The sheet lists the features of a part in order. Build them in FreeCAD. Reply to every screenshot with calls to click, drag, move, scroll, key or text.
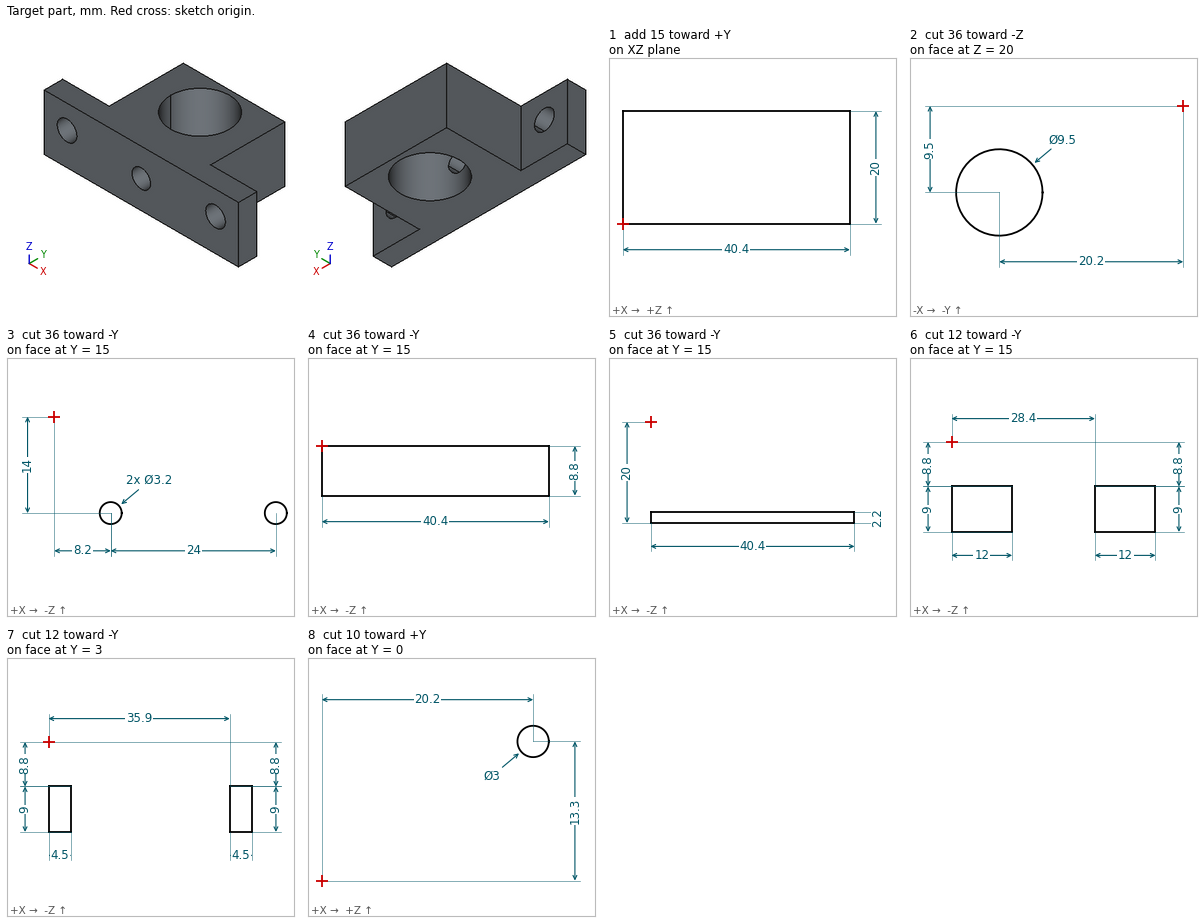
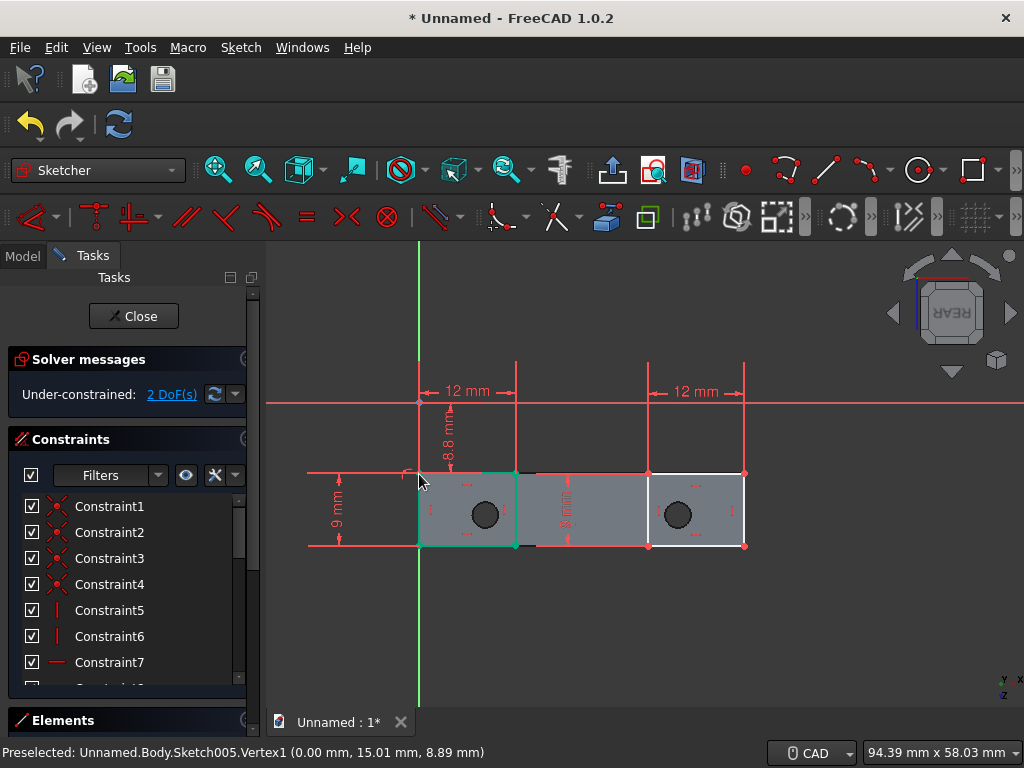
click(648, 474)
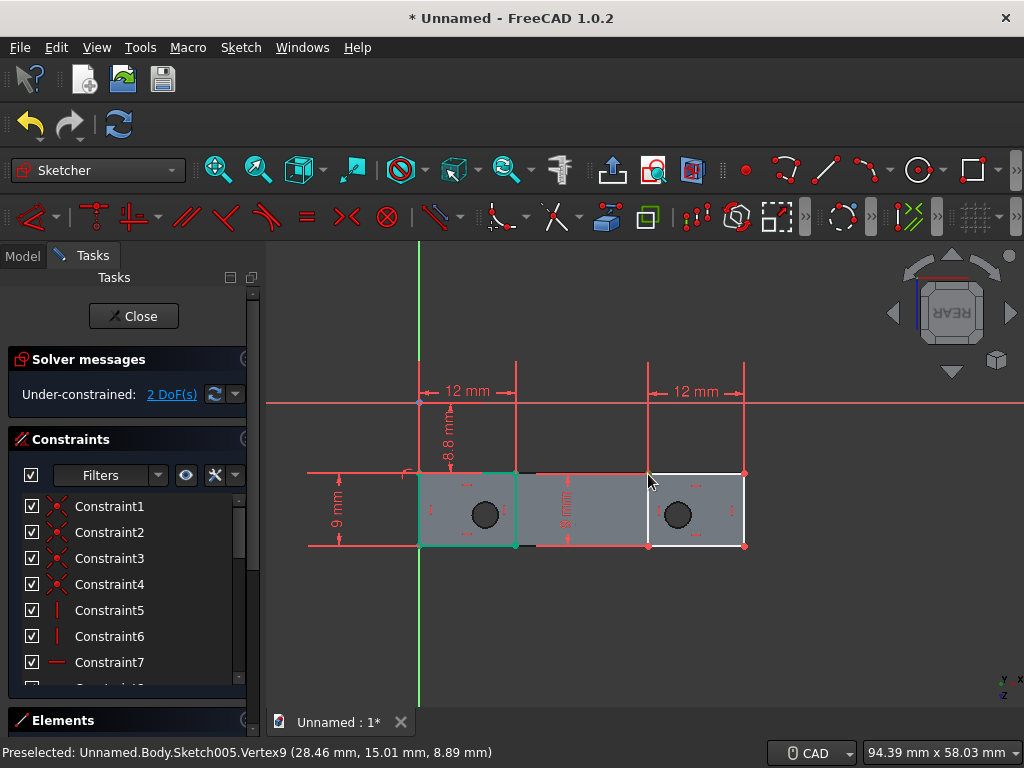
key(i)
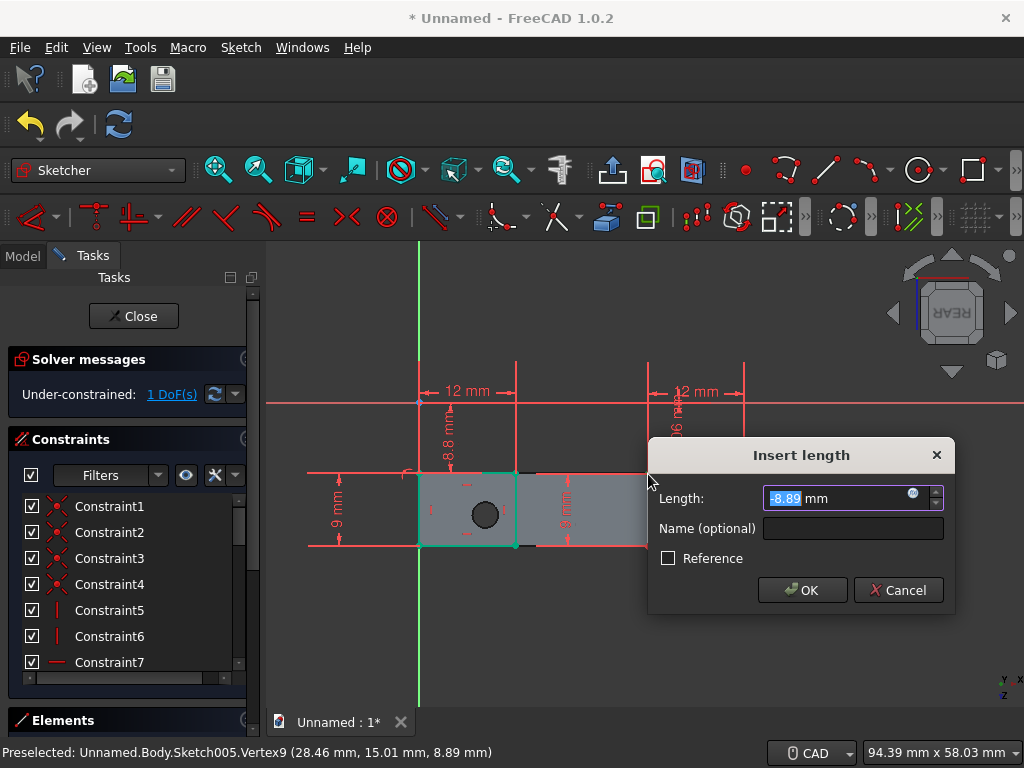
text(-8.8)
key(Return)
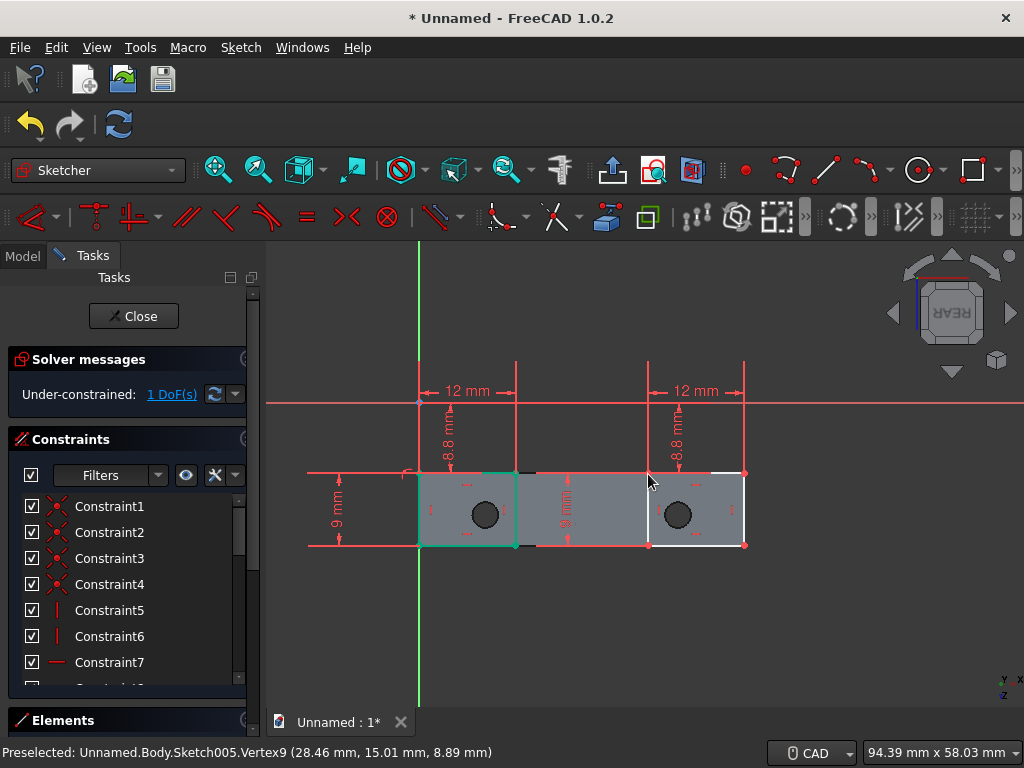
click(648, 473)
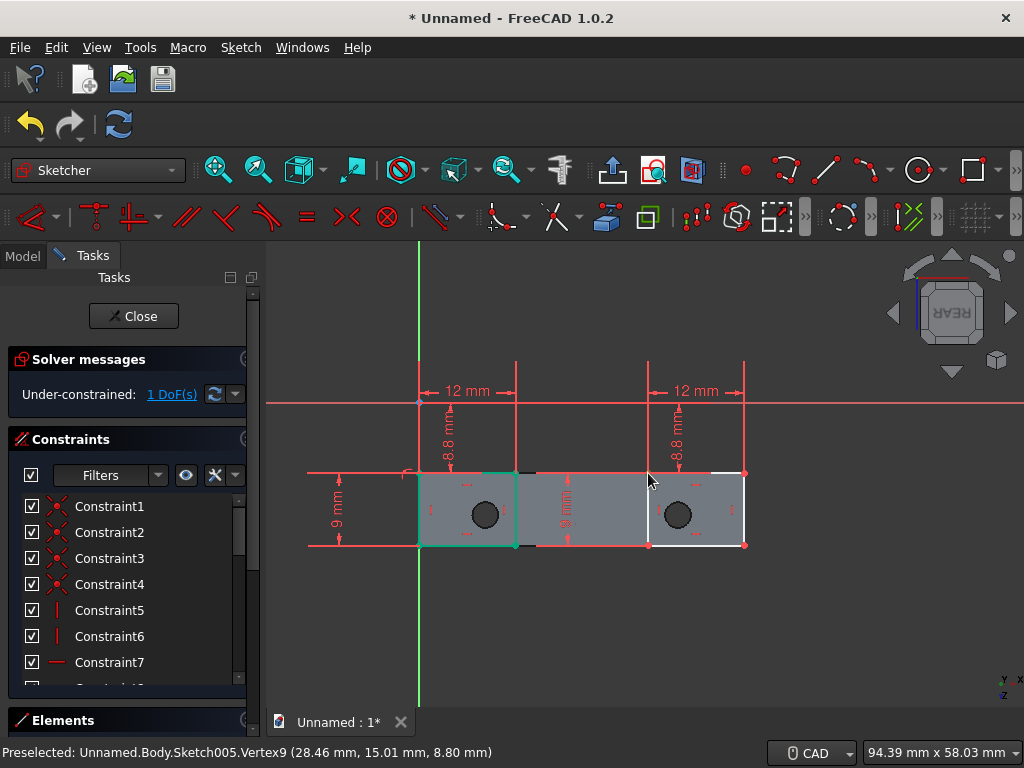
key(l)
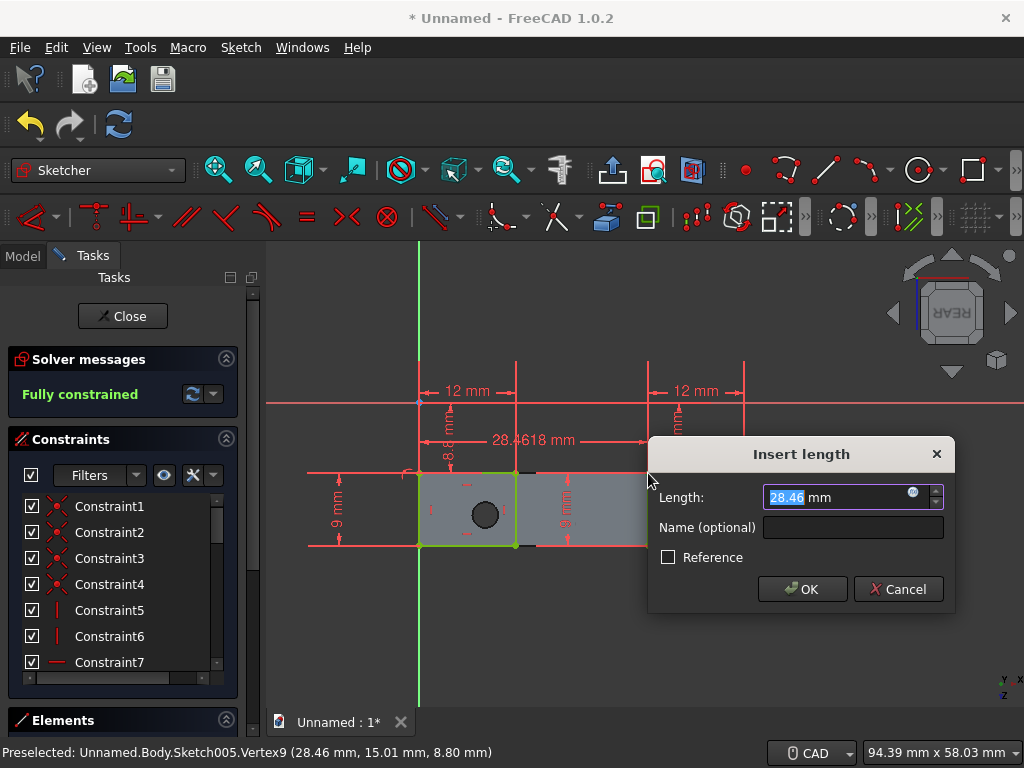
text(28.4)
key(Return)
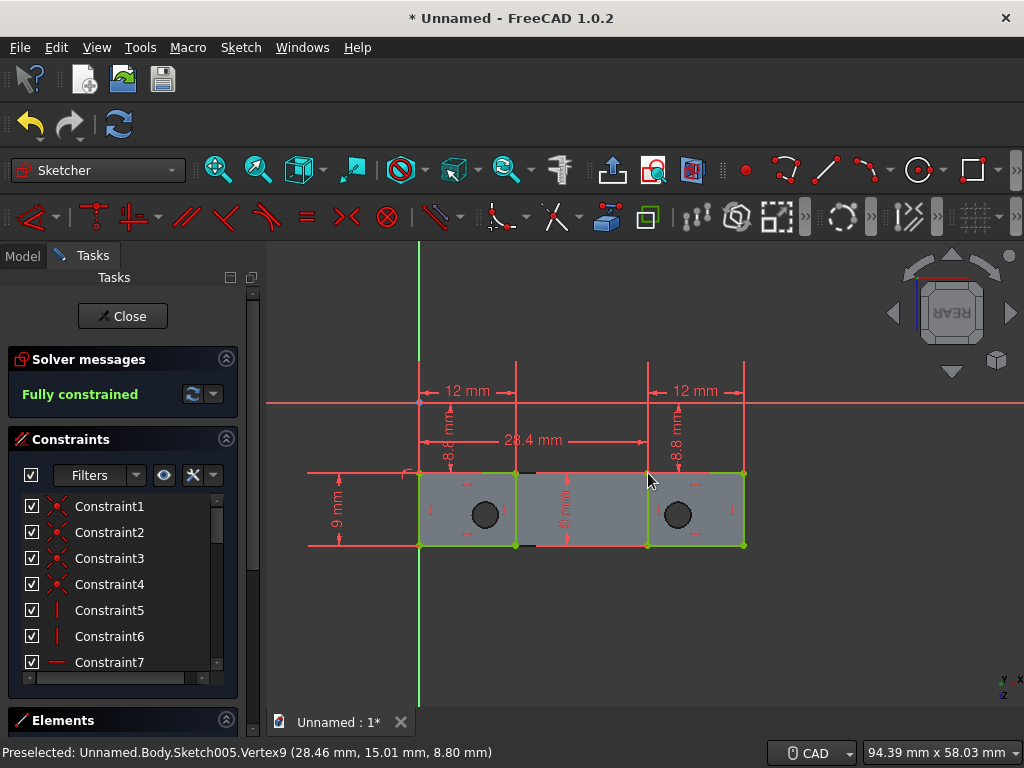
click(123, 316)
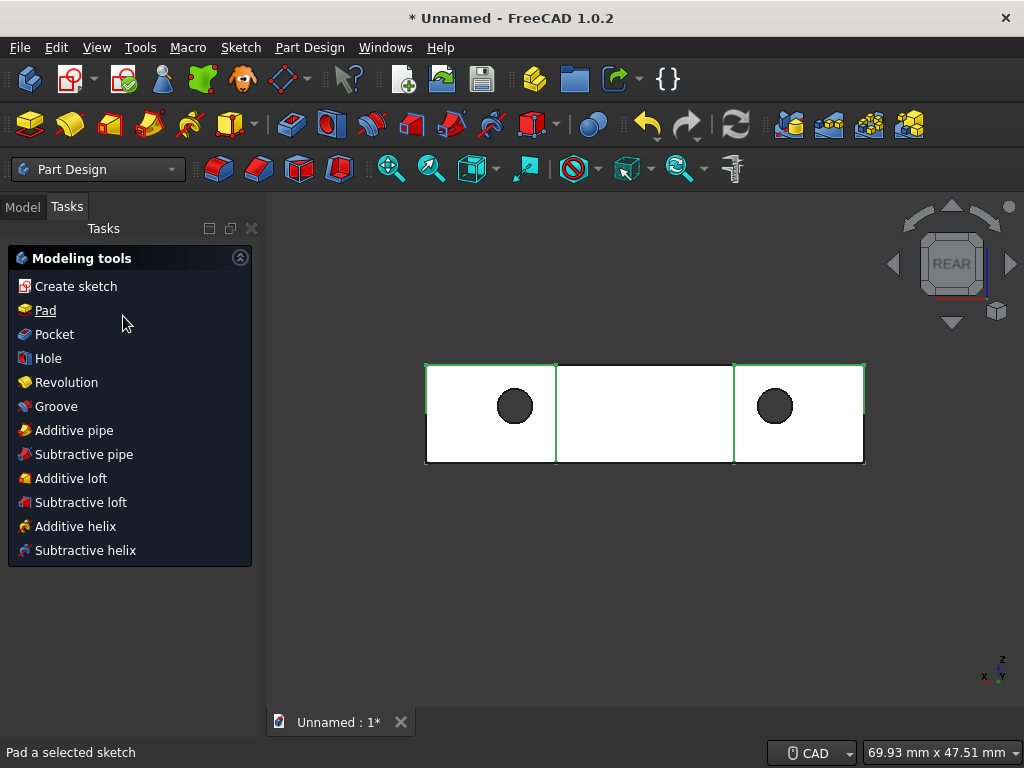
click(292, 124)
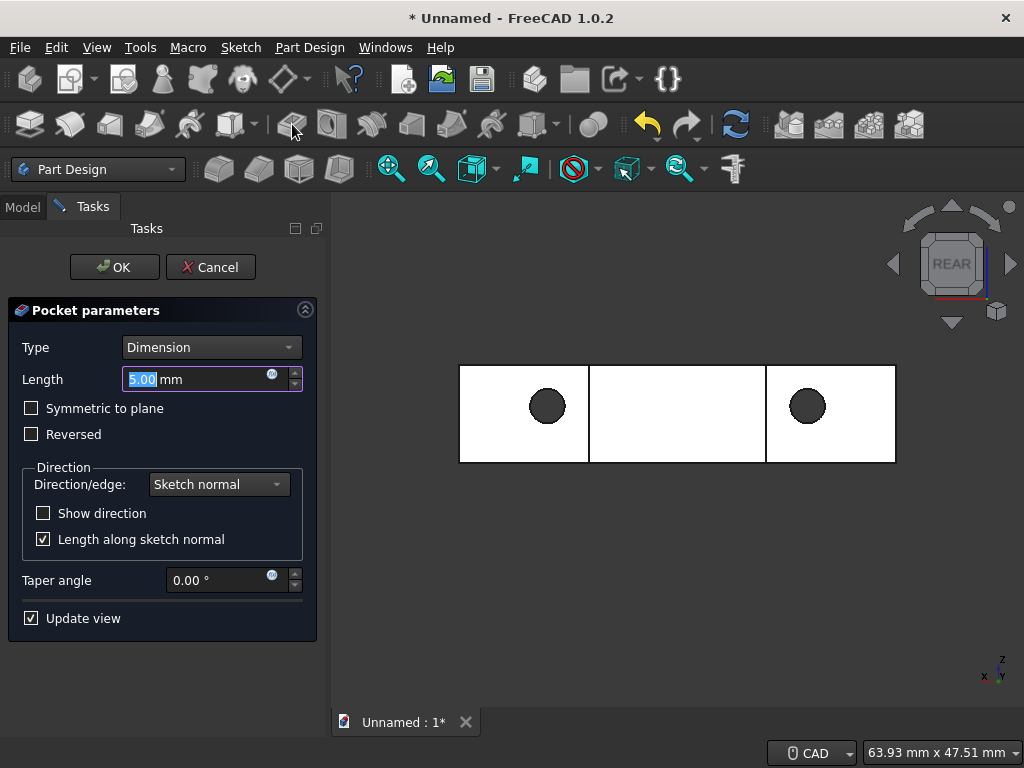
text(12)
key(Tab)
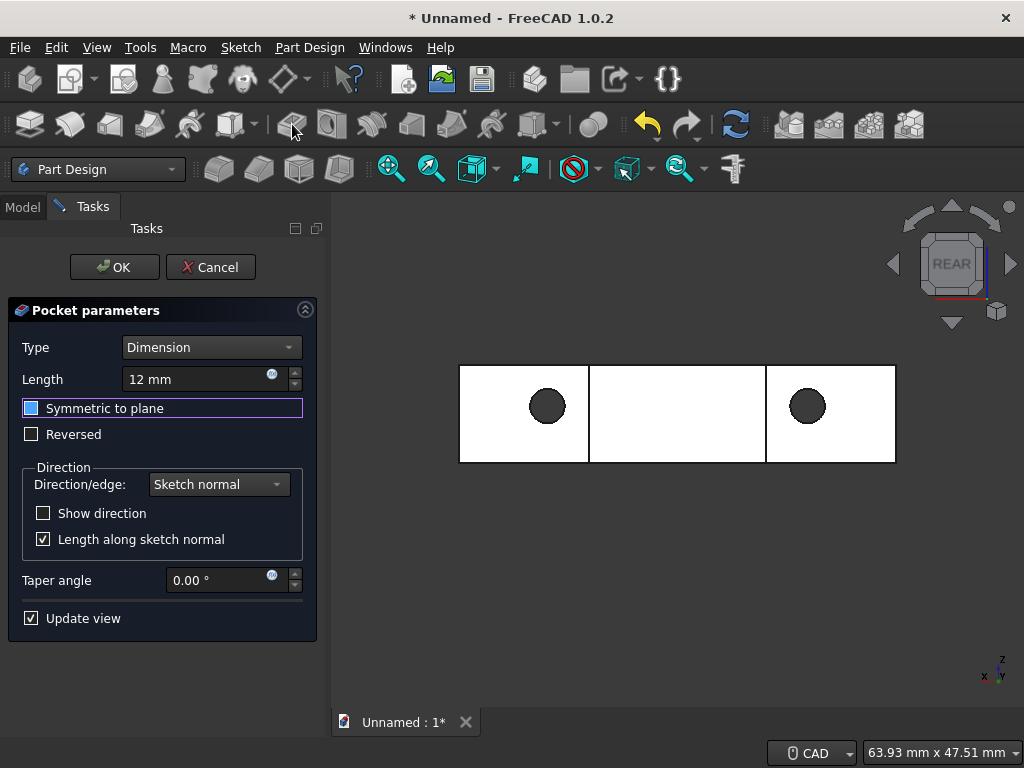
click(115, 267)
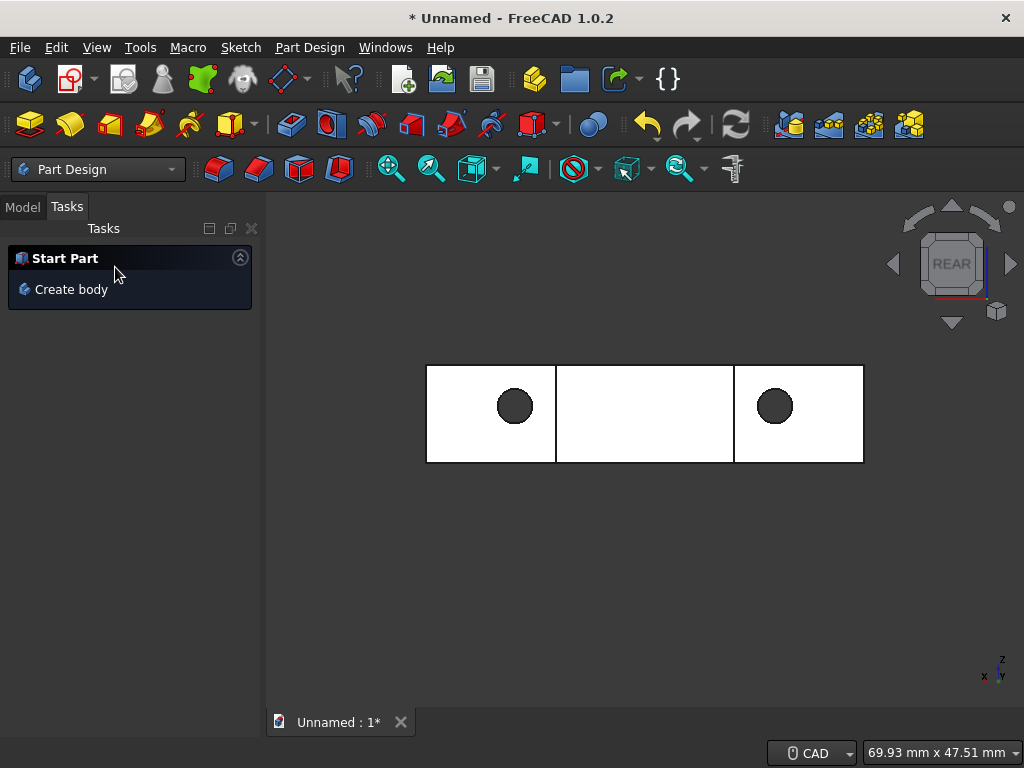
click(818, 427)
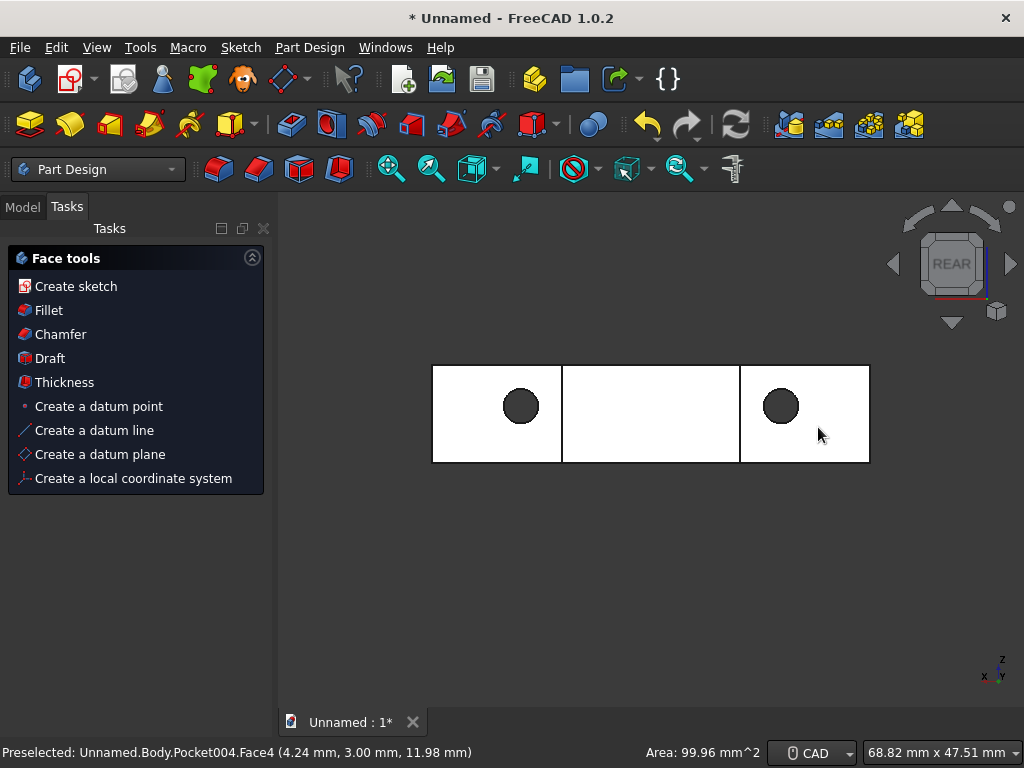
click(70, 80)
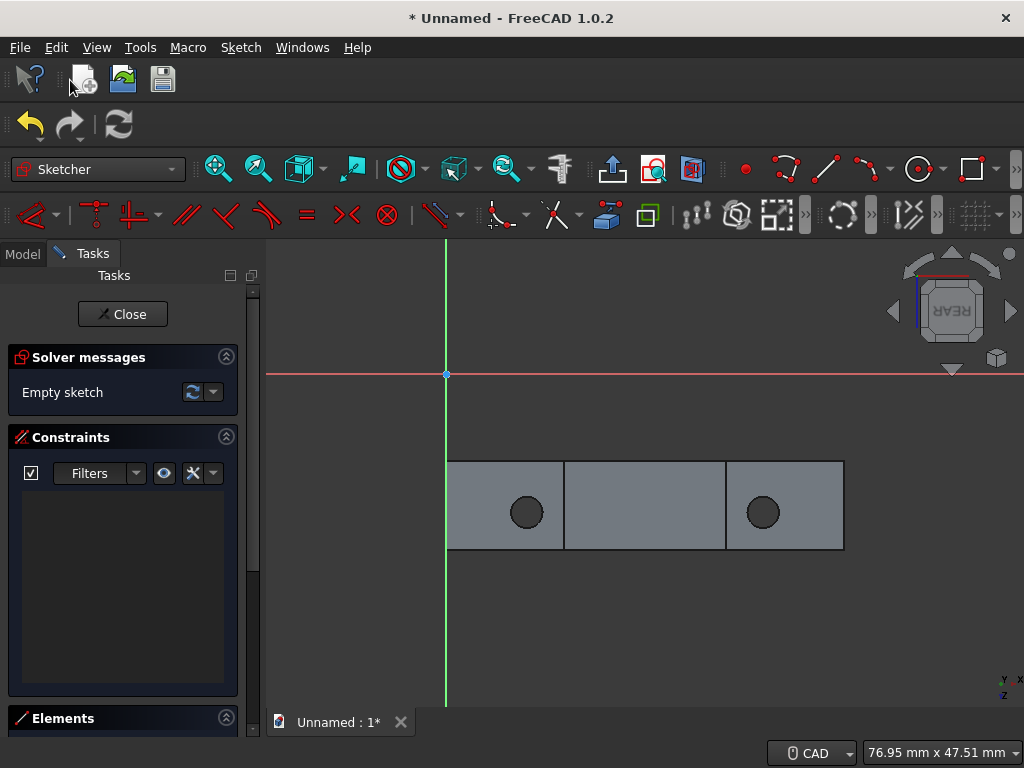
click(694, 170)